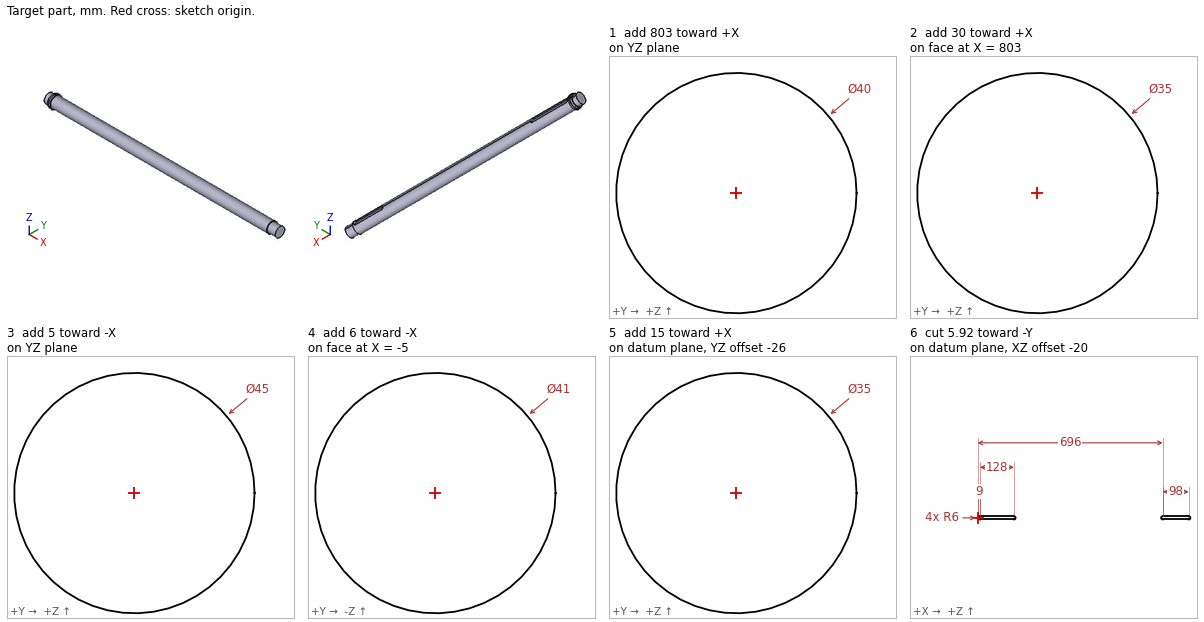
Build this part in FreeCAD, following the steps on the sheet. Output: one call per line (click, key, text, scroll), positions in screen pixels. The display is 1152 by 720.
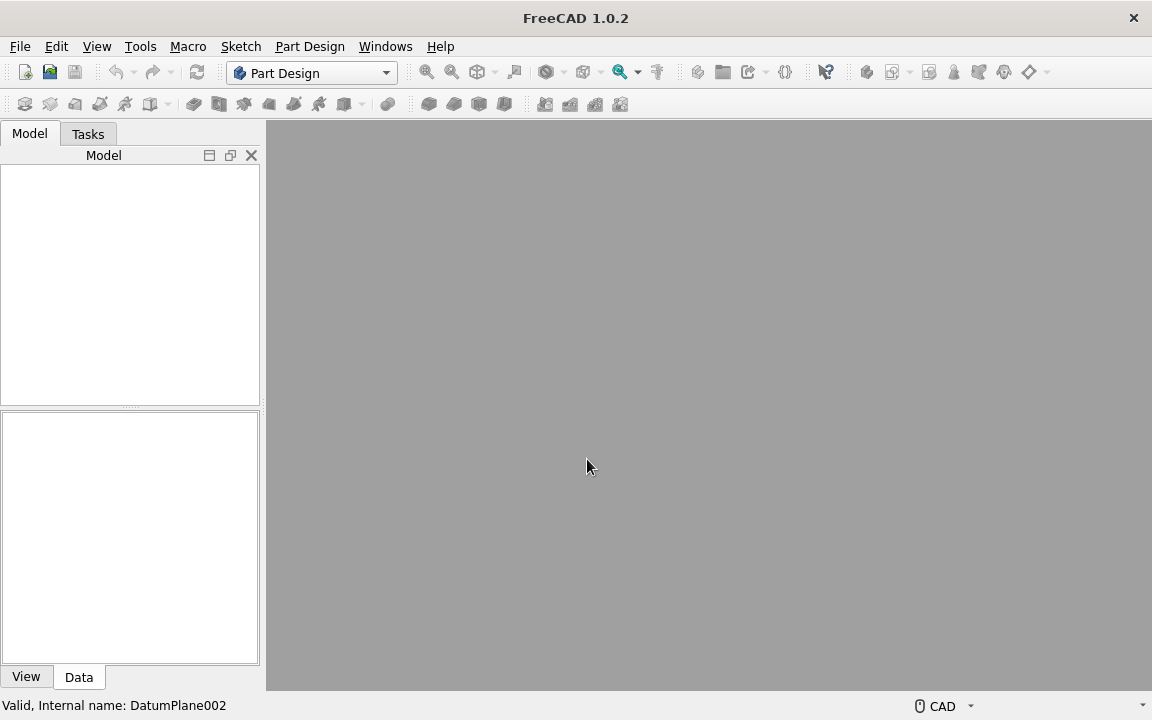
click(25, 72)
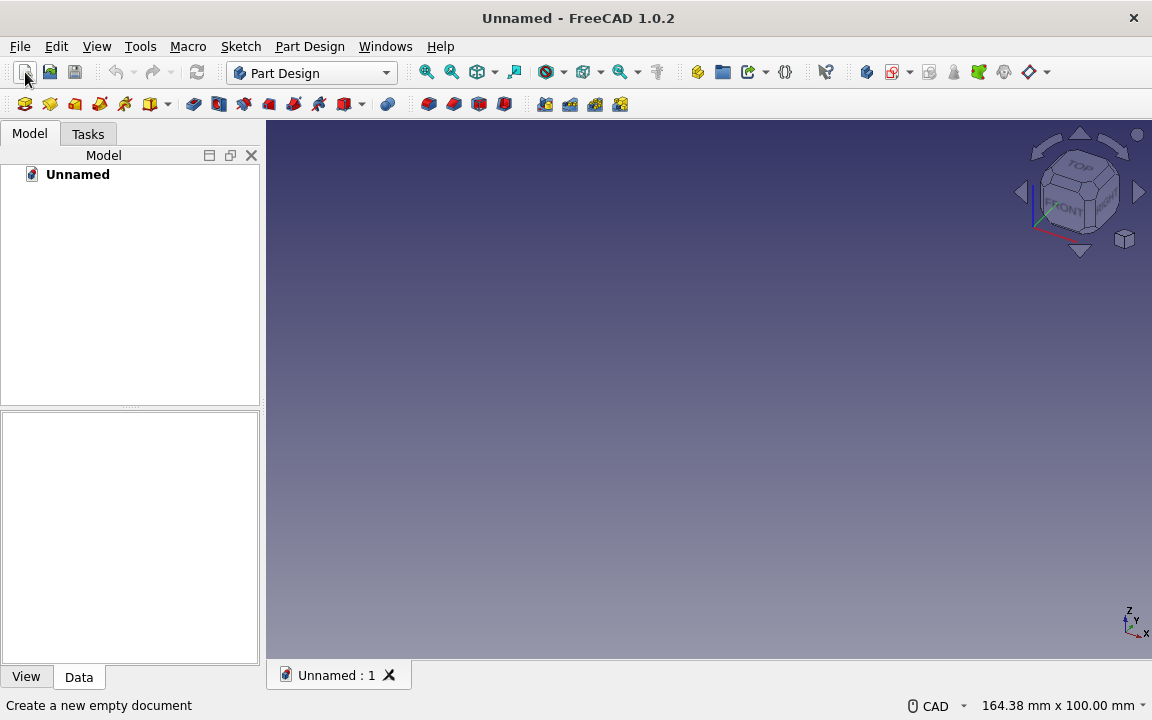
click(892, 72)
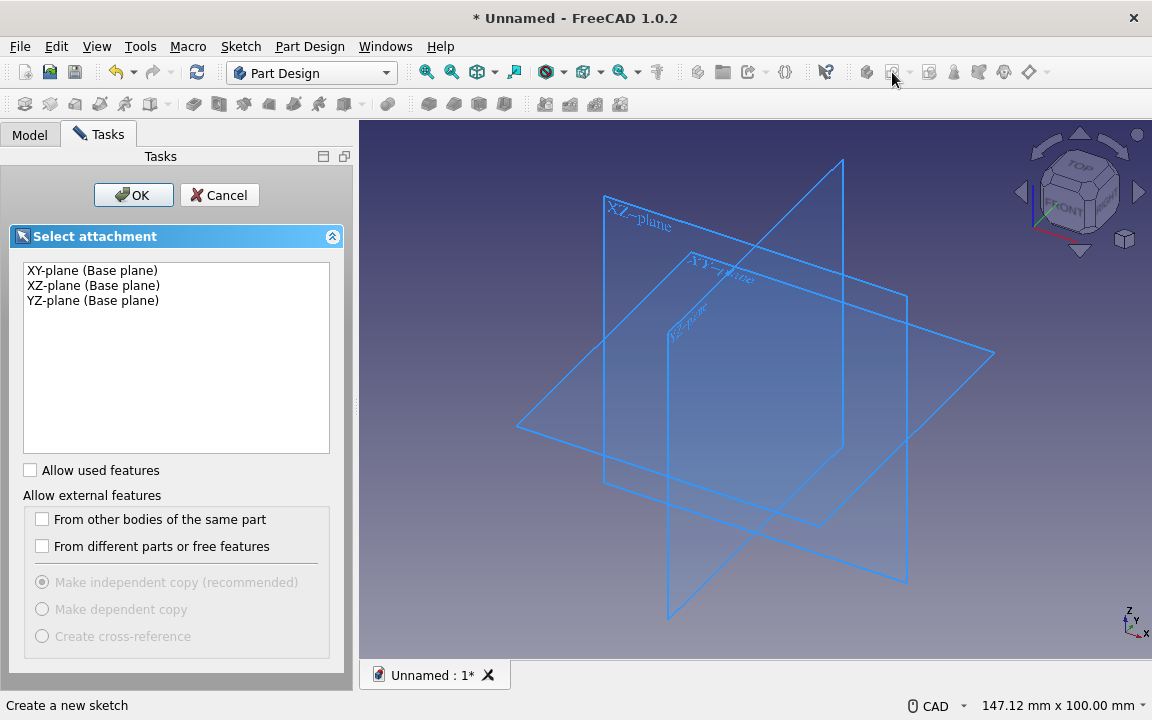
click(84, 300)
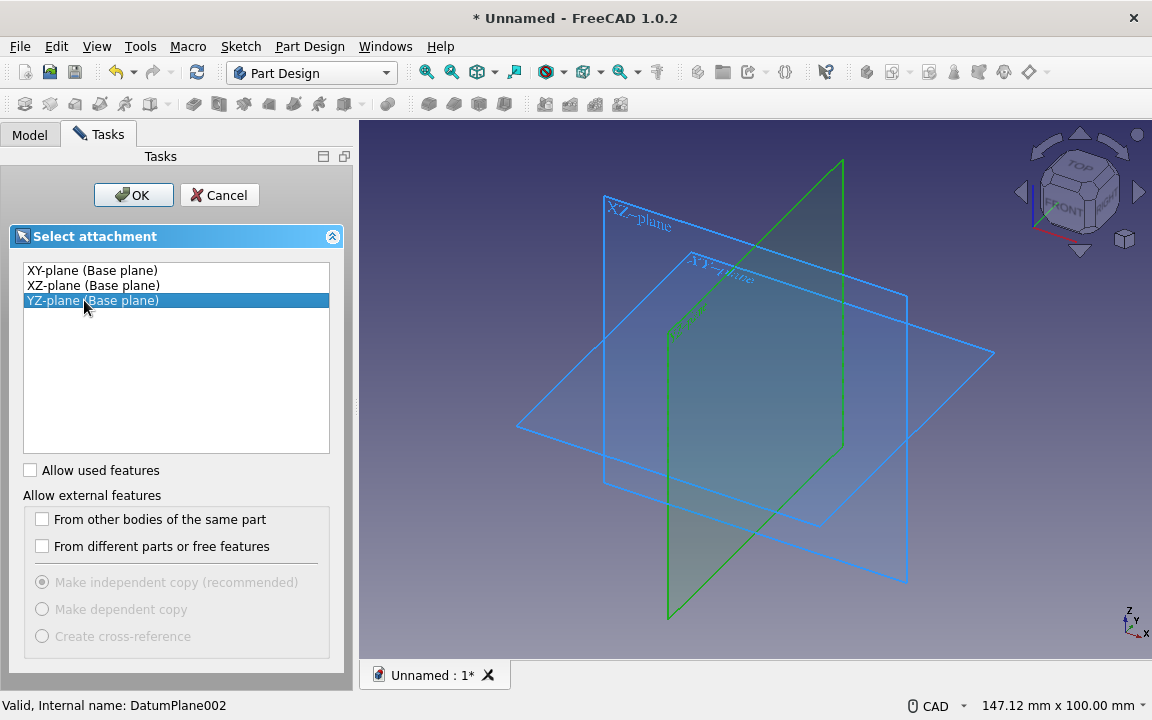
click(134, 195)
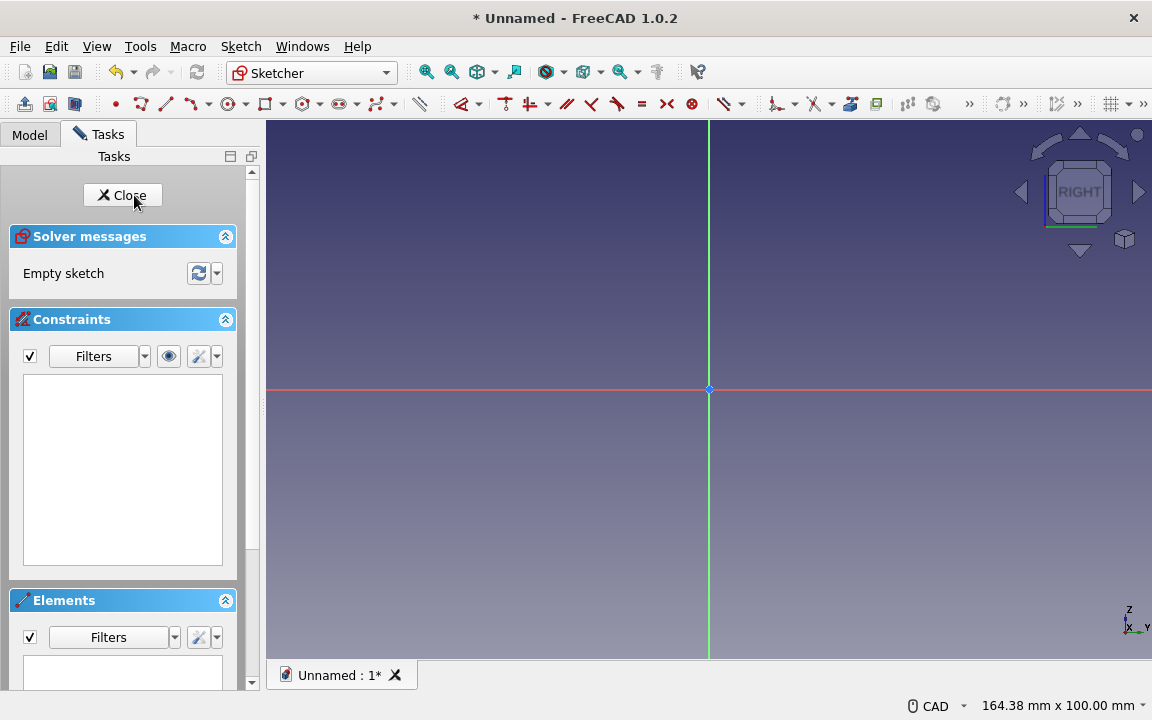
scroll(848, 390, up, 2)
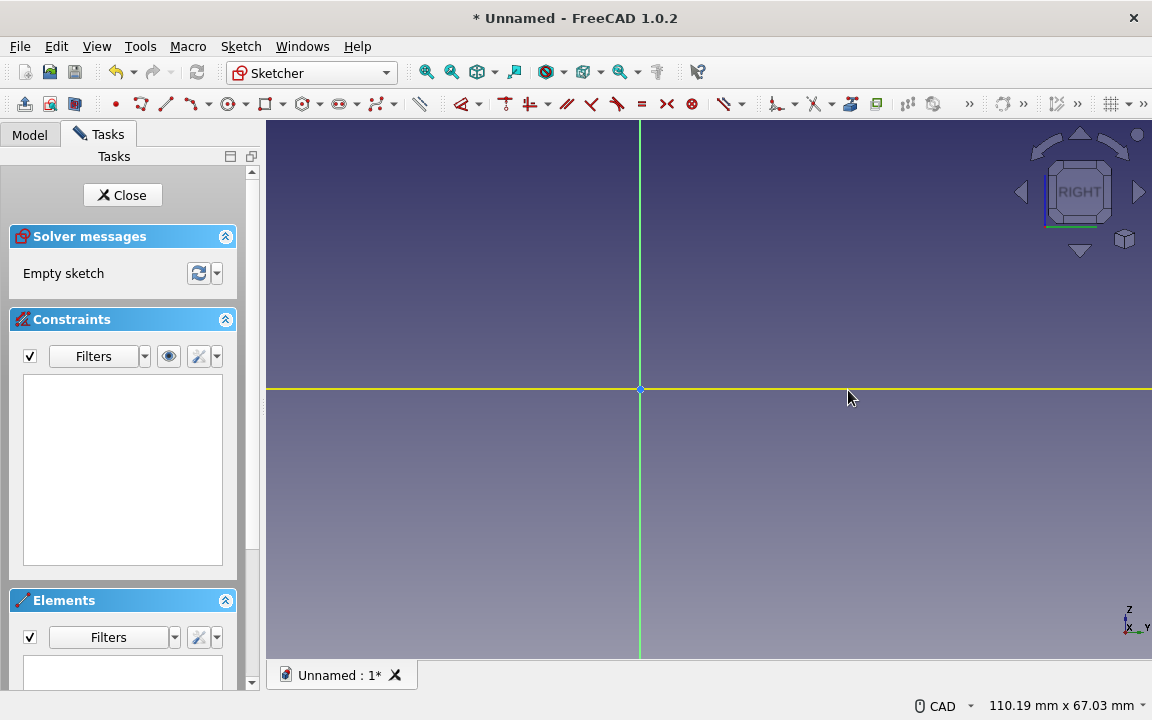
click(228, 104)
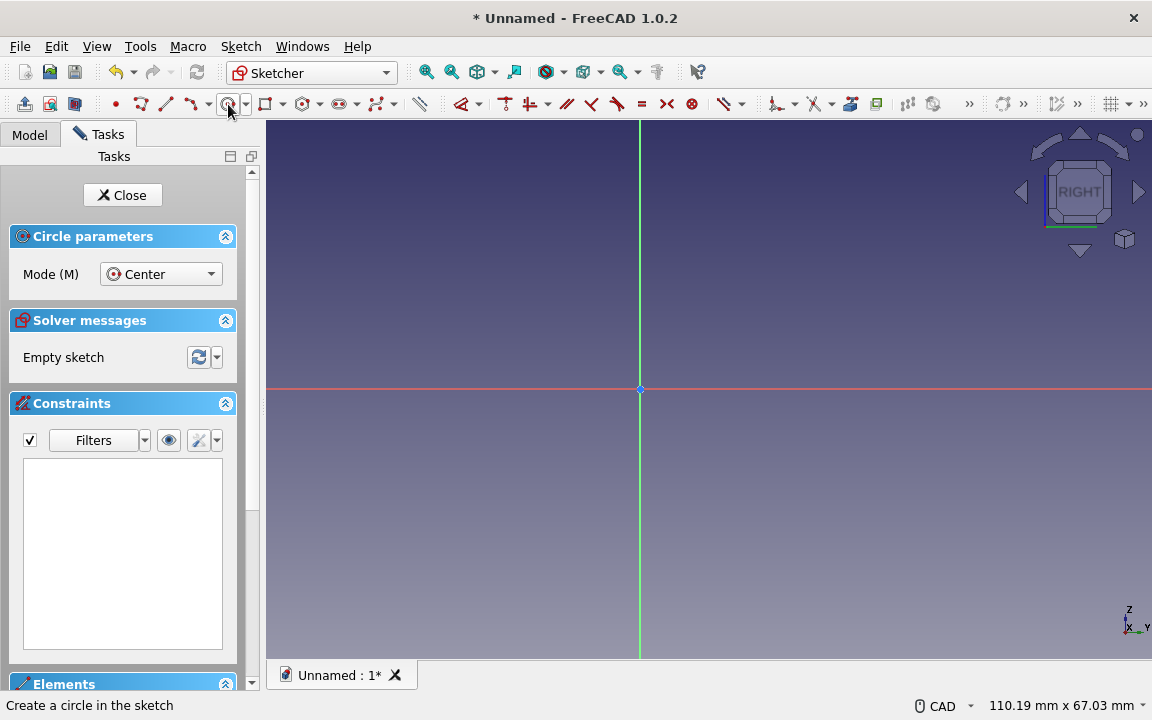
click(640, 389)
move(754, 275)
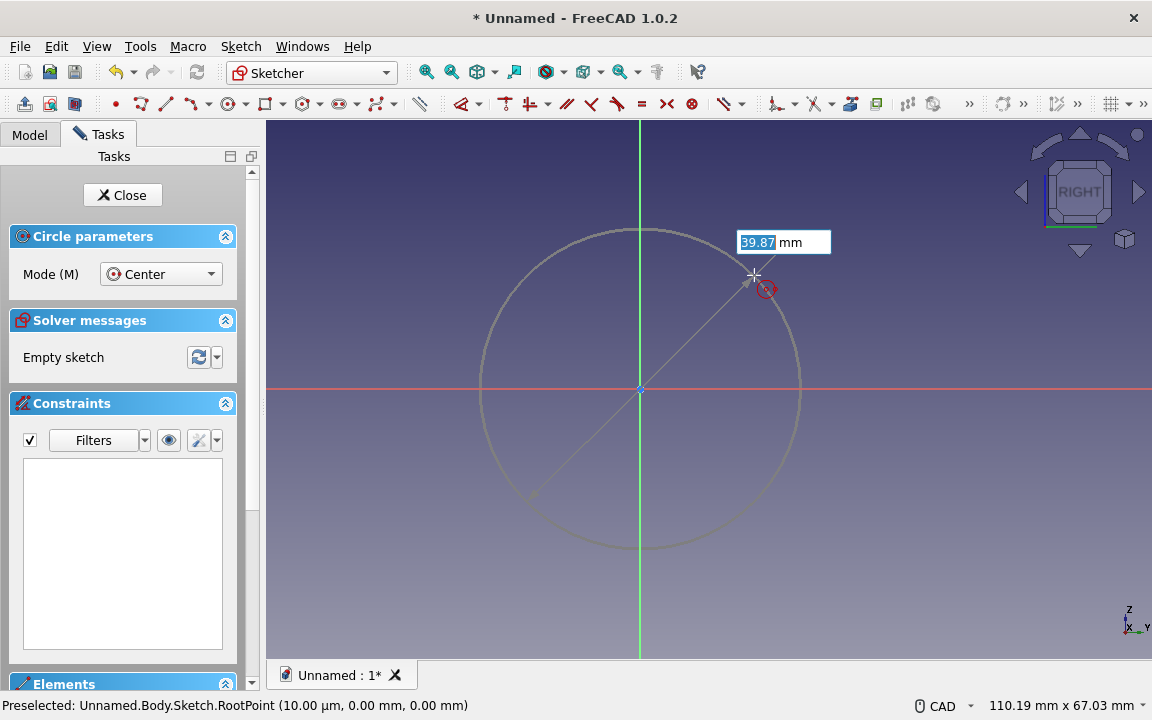
text(40)
key(Return)
key(Escape)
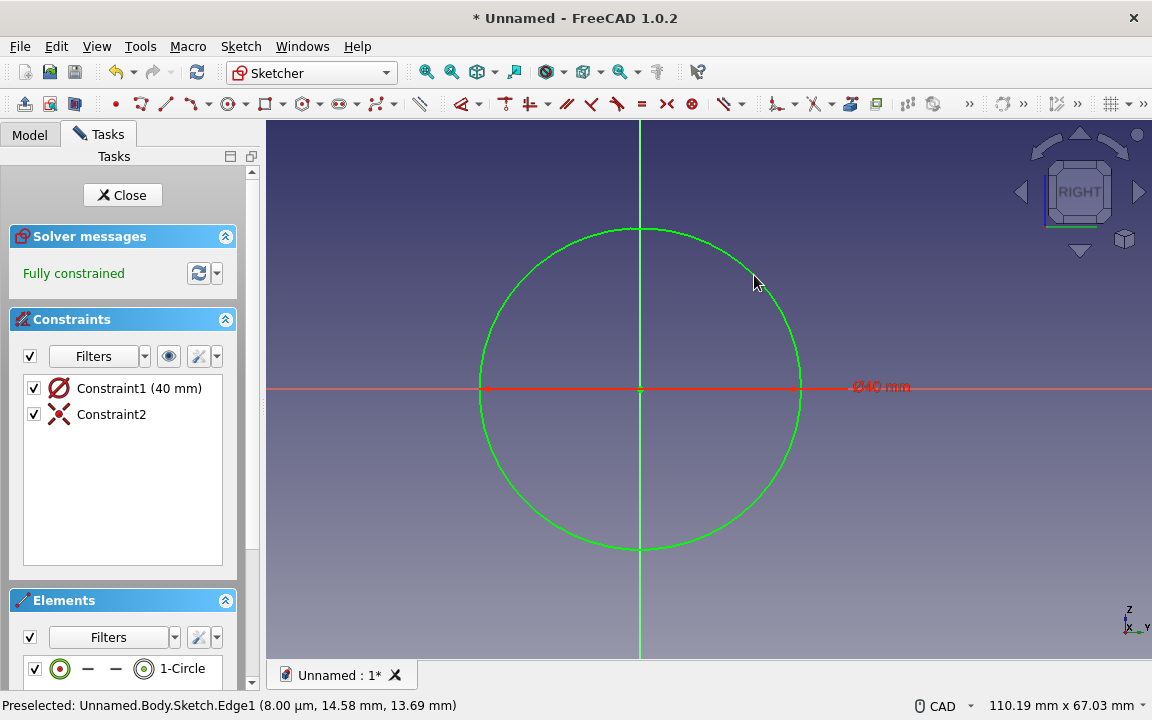
click(123, 195)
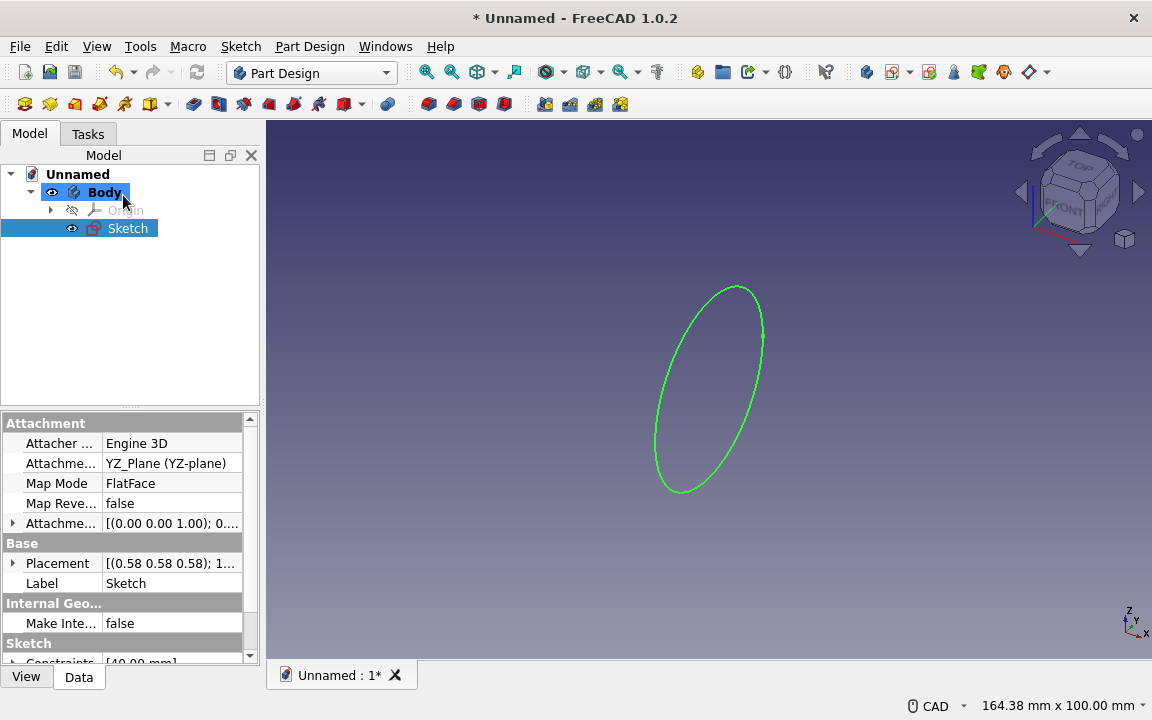
click(25, 104)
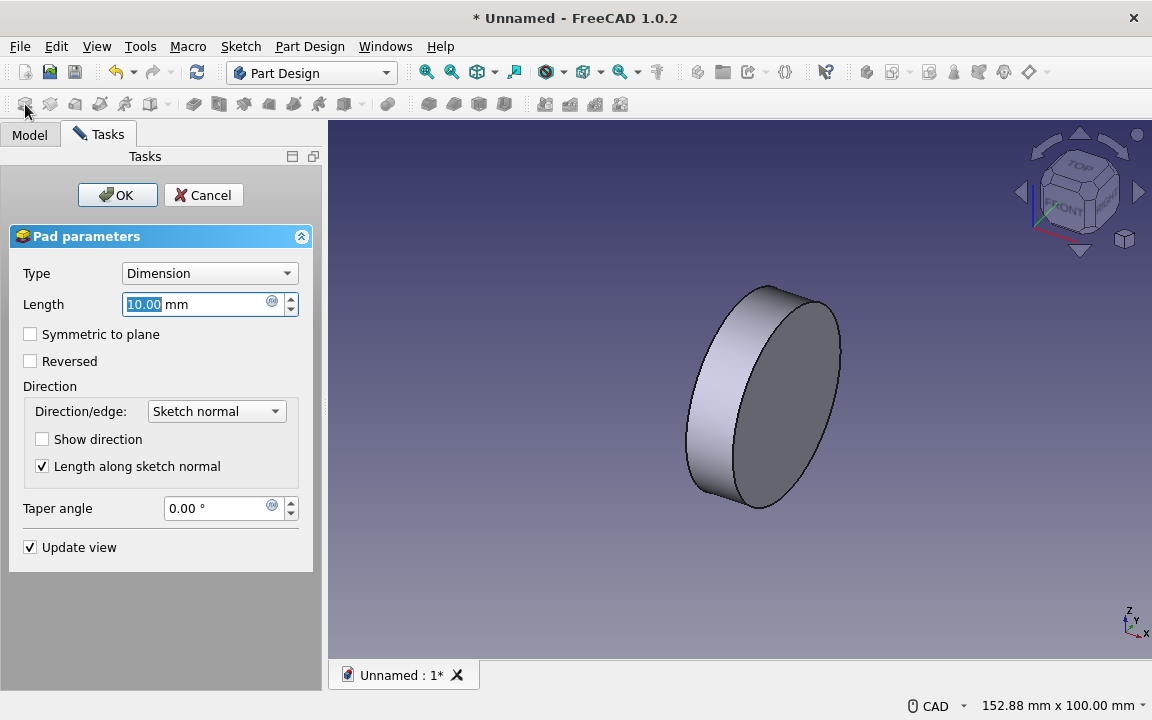
text(803)
key(Tab)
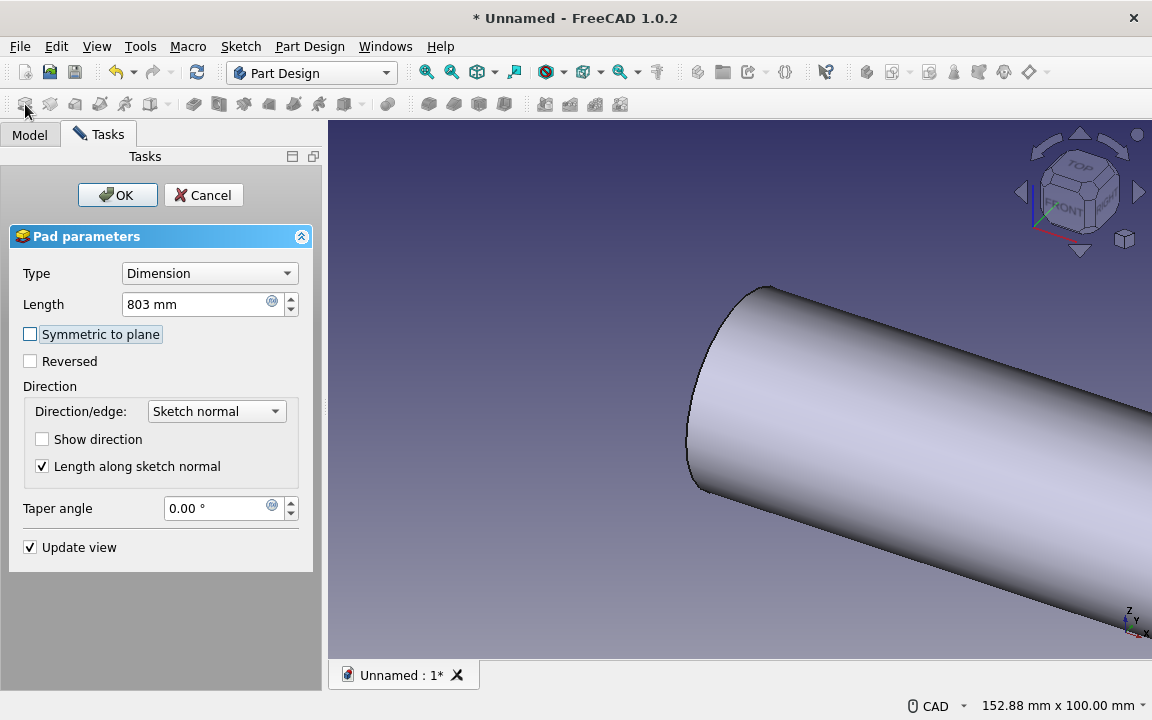
click(118, 195)